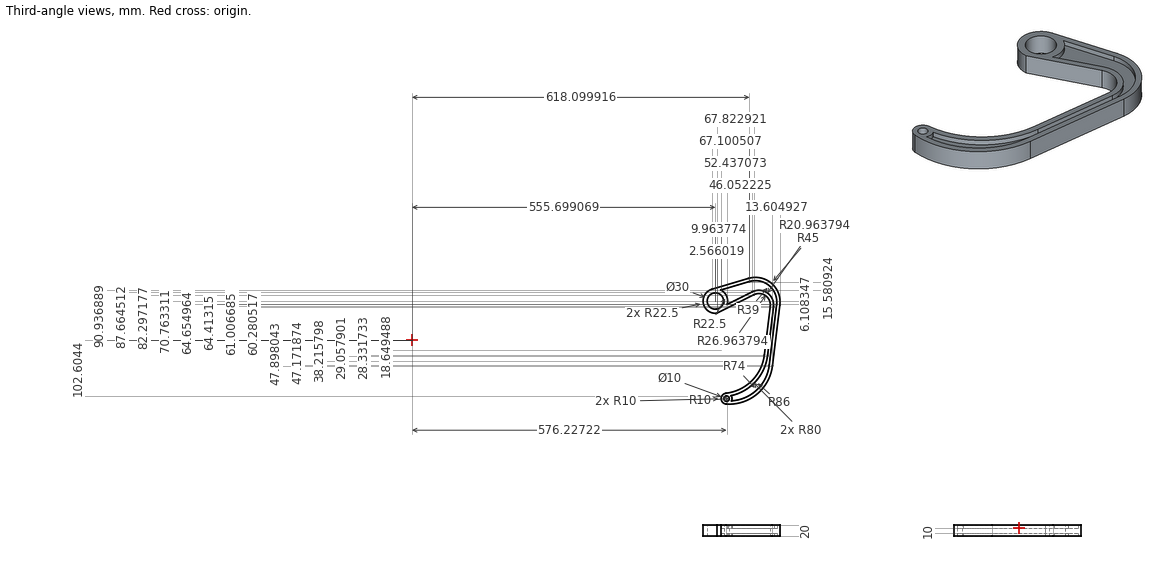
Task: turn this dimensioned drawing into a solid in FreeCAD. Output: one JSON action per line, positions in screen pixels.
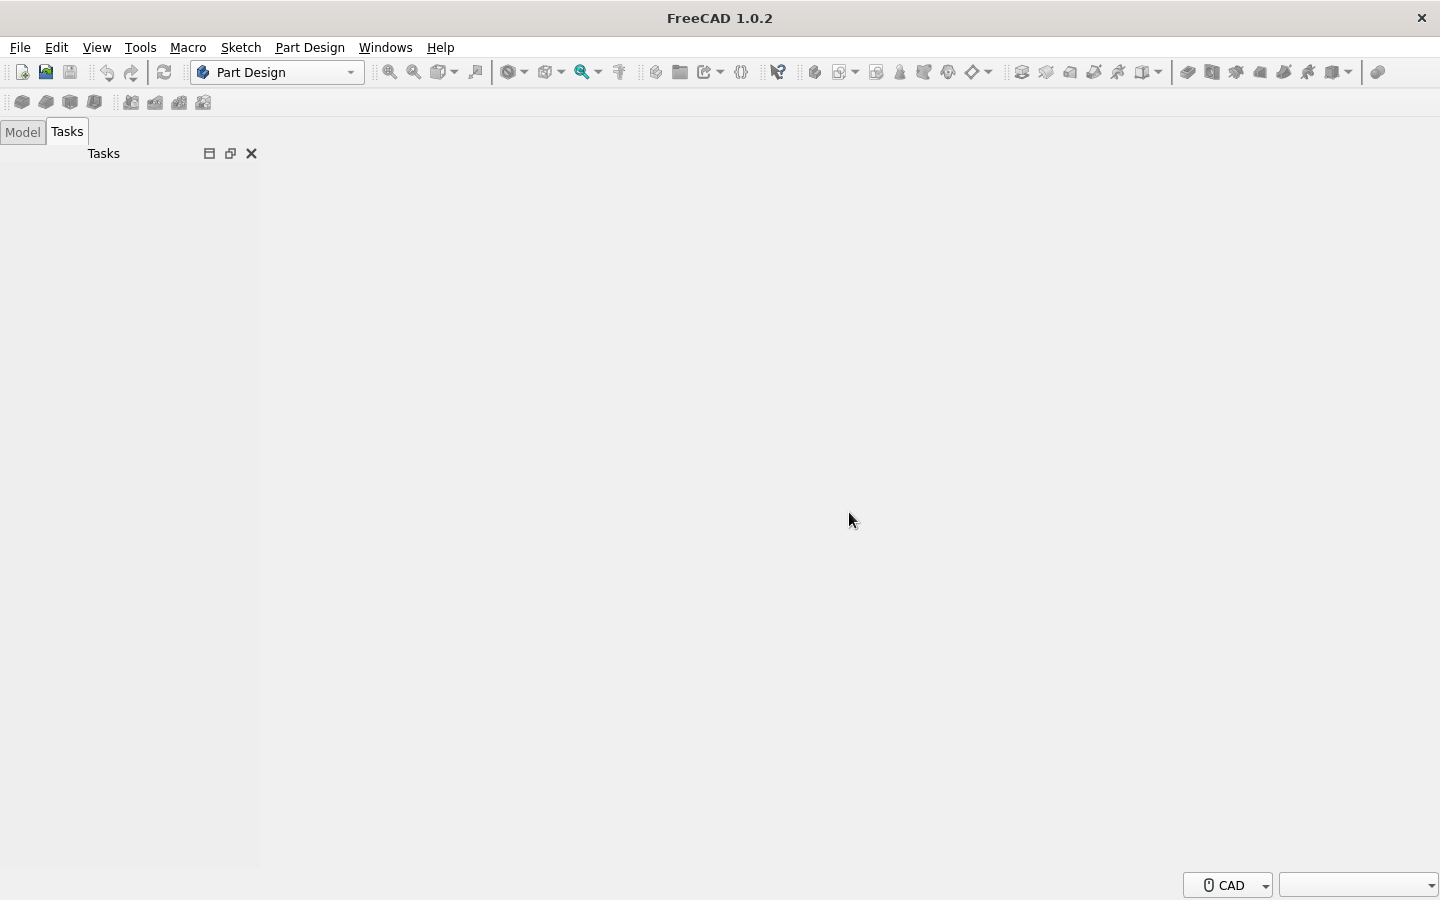
{"action": "left_click", "coordinate": [22, 72]}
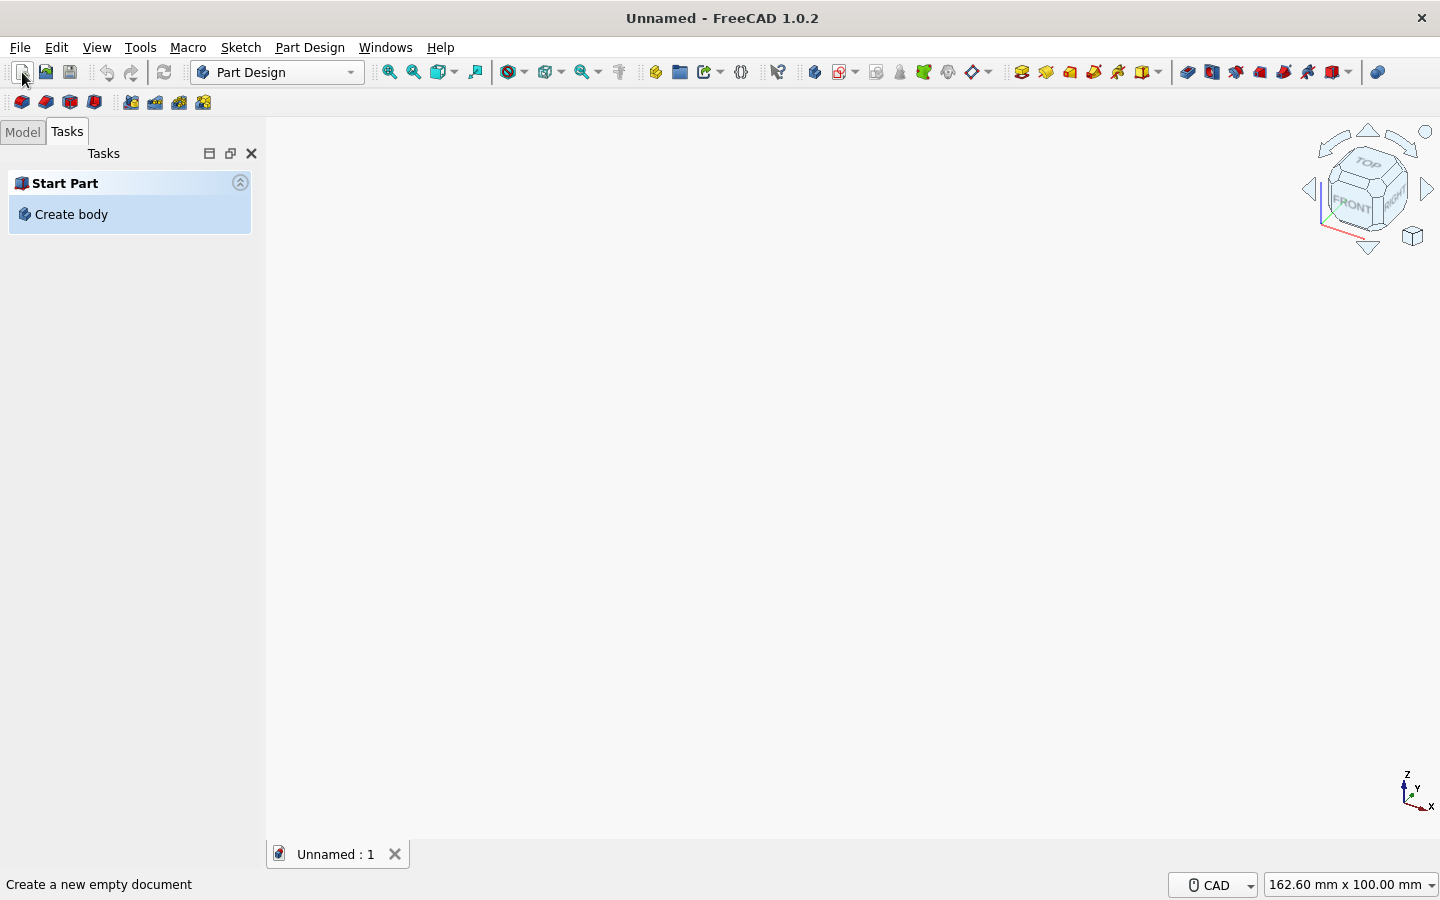
{"action": "left_click", "coordinate": [840, 72]}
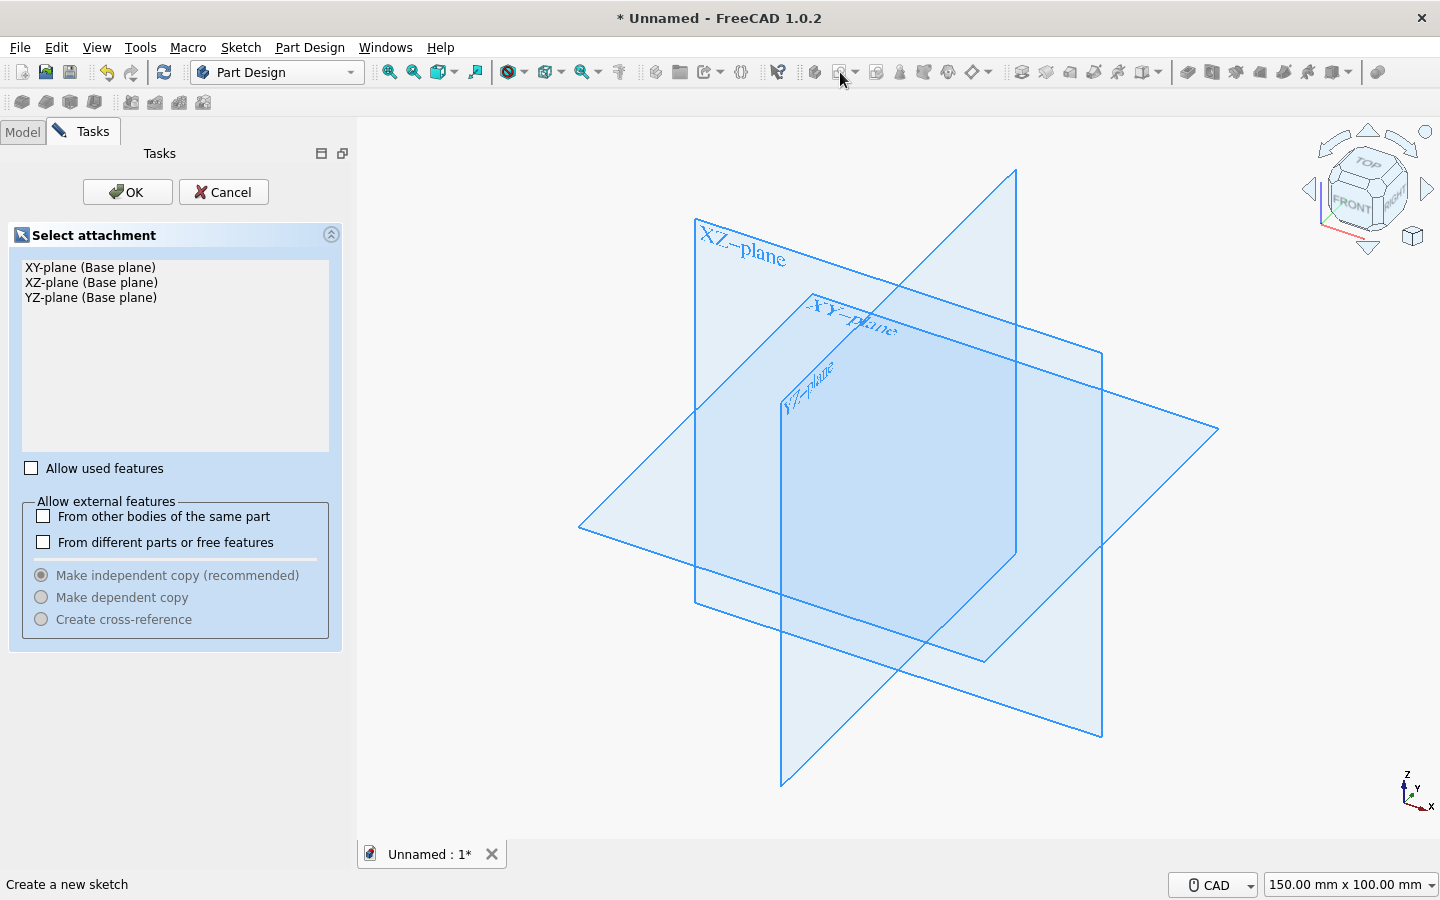
{"action": "left_click", "coordinate": [82, 268]}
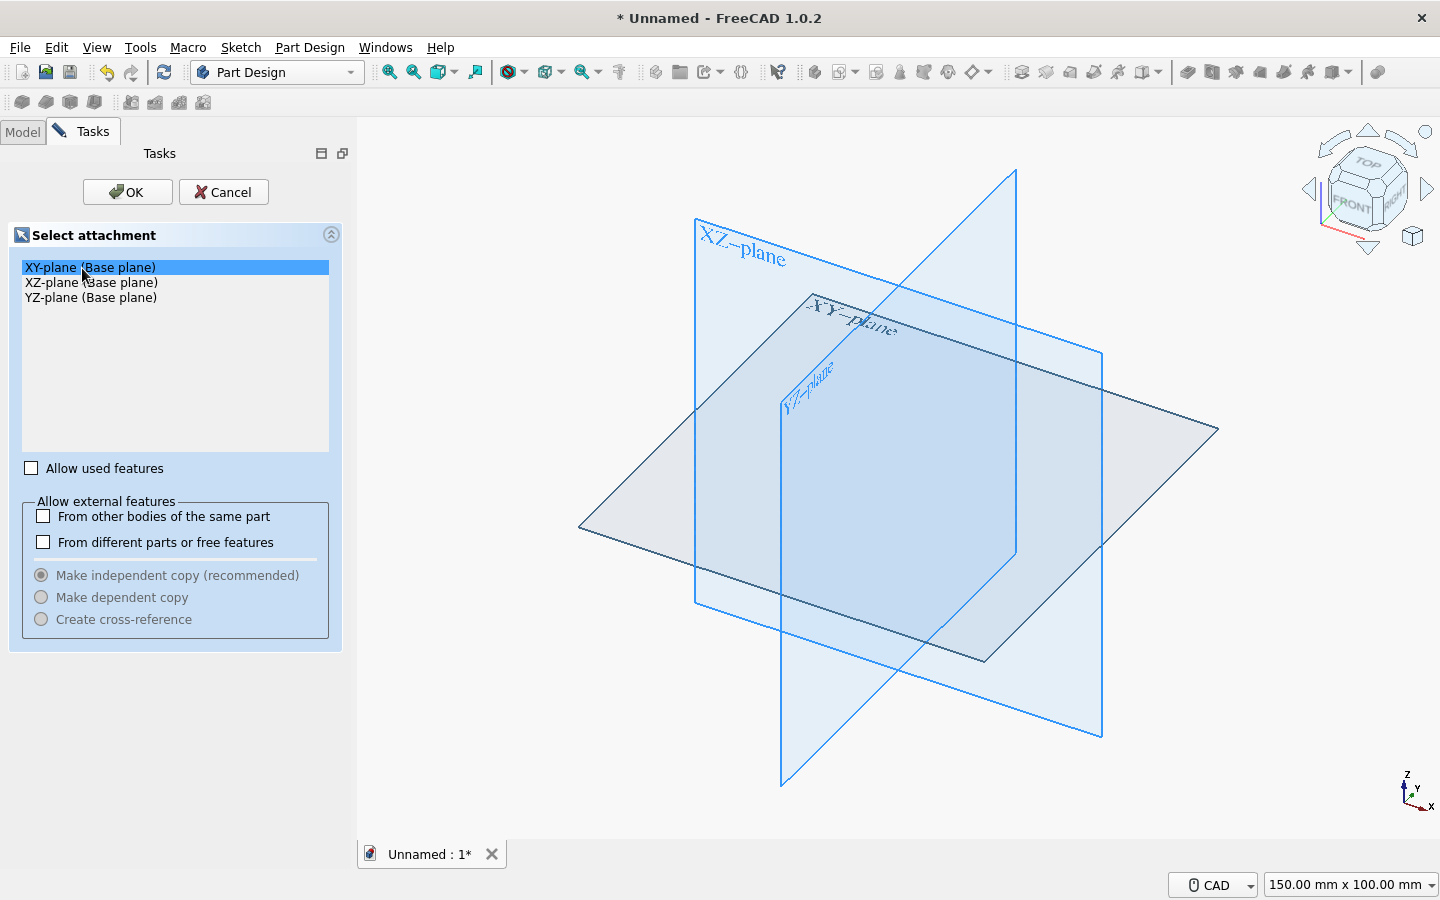
{"action": "left_click", "coordinate": [128, 192]}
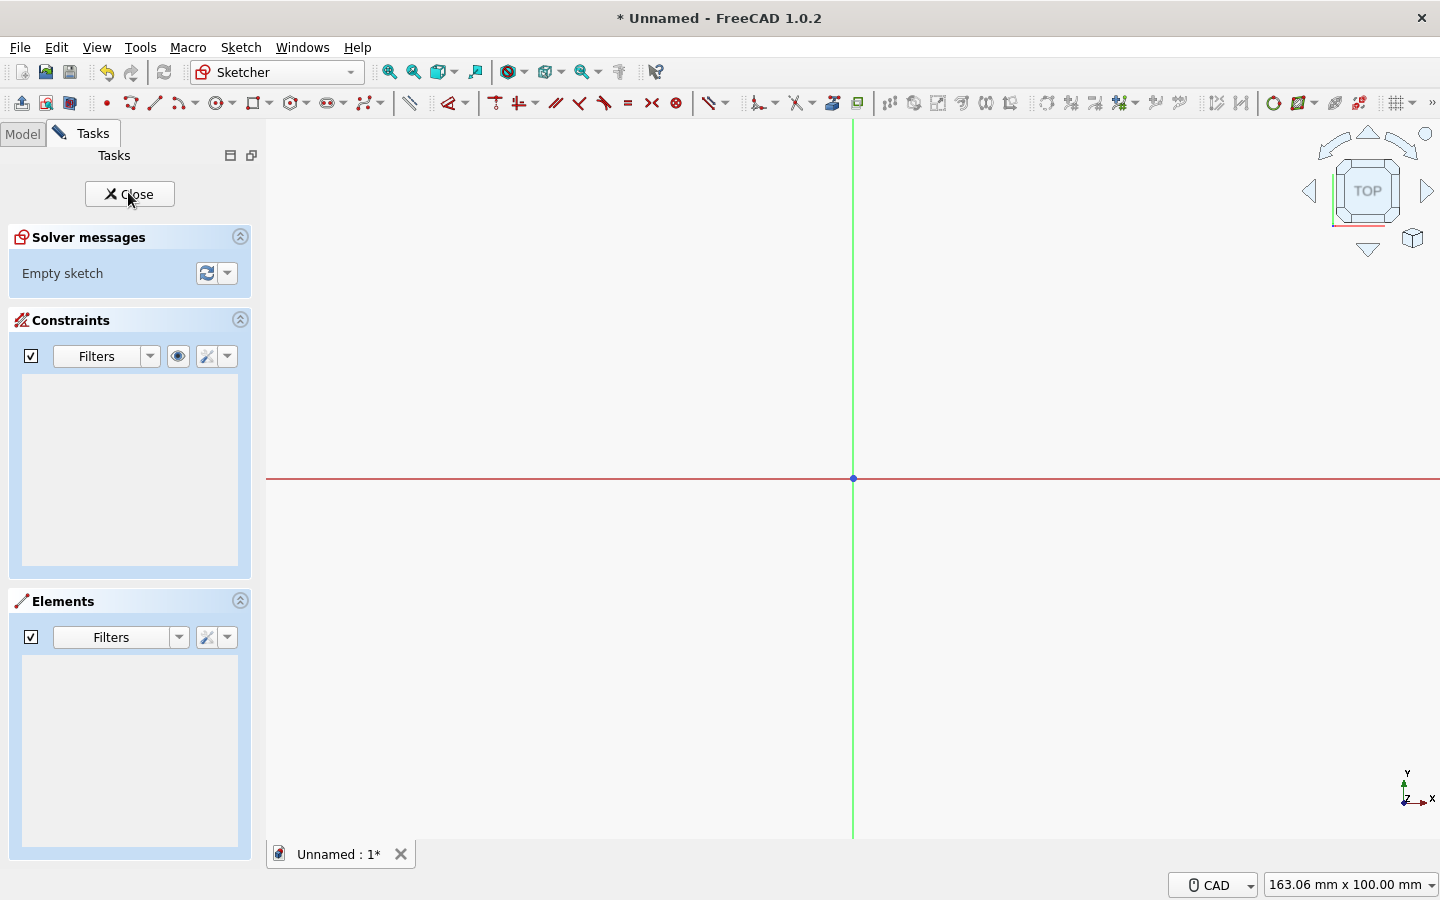
{"action": "scroll", "coordinate": [294, 475], "scroll_direction": "down", "scroll_amount": 9}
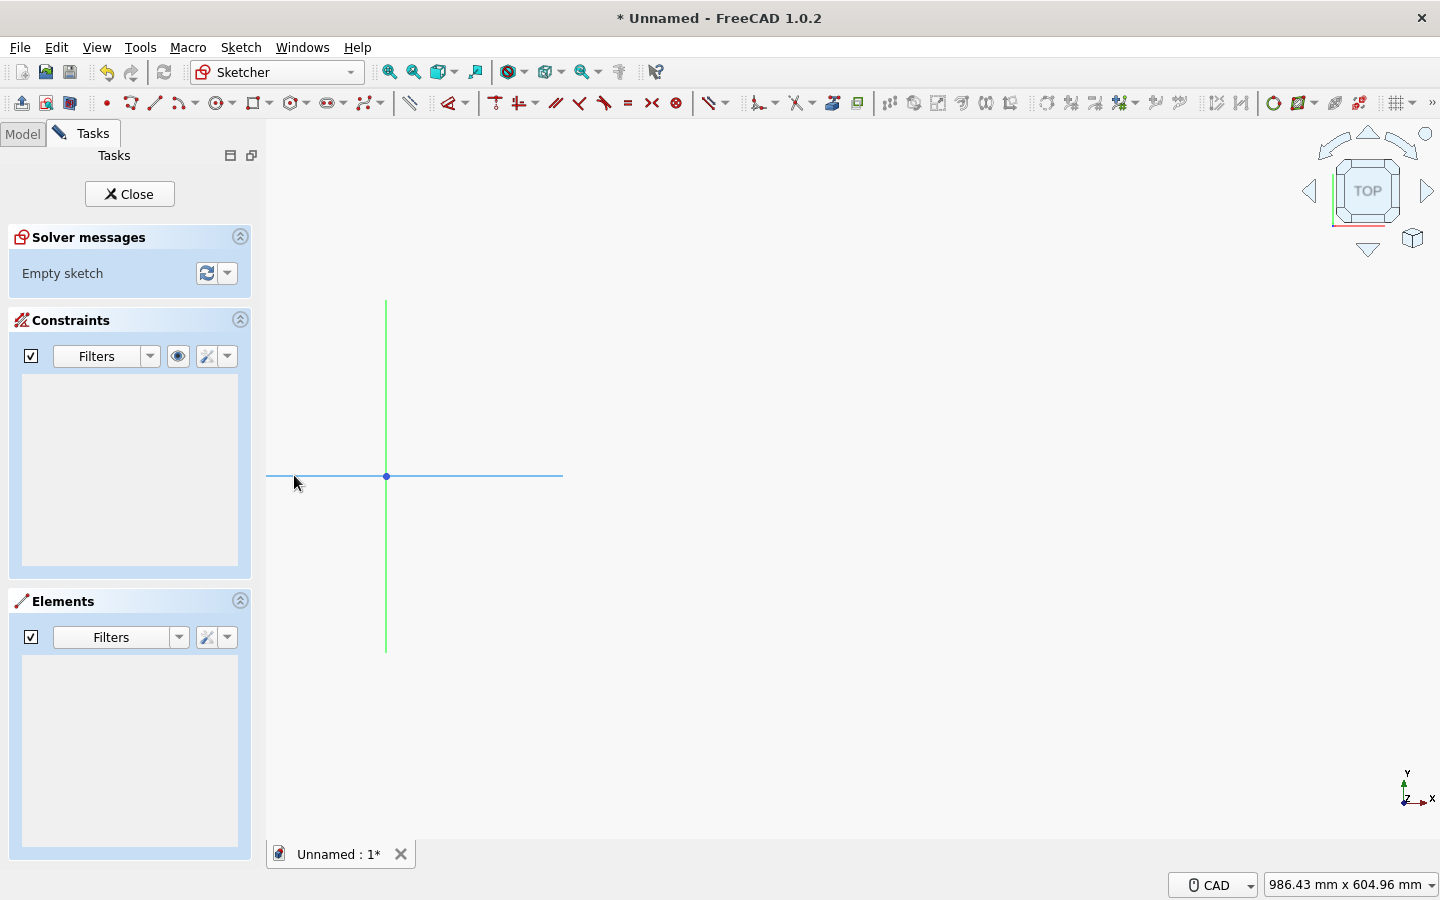
{"action": "scroll", "coordinate": [1275, 480], "scroll_direction": "up", "scroll_amount": 3}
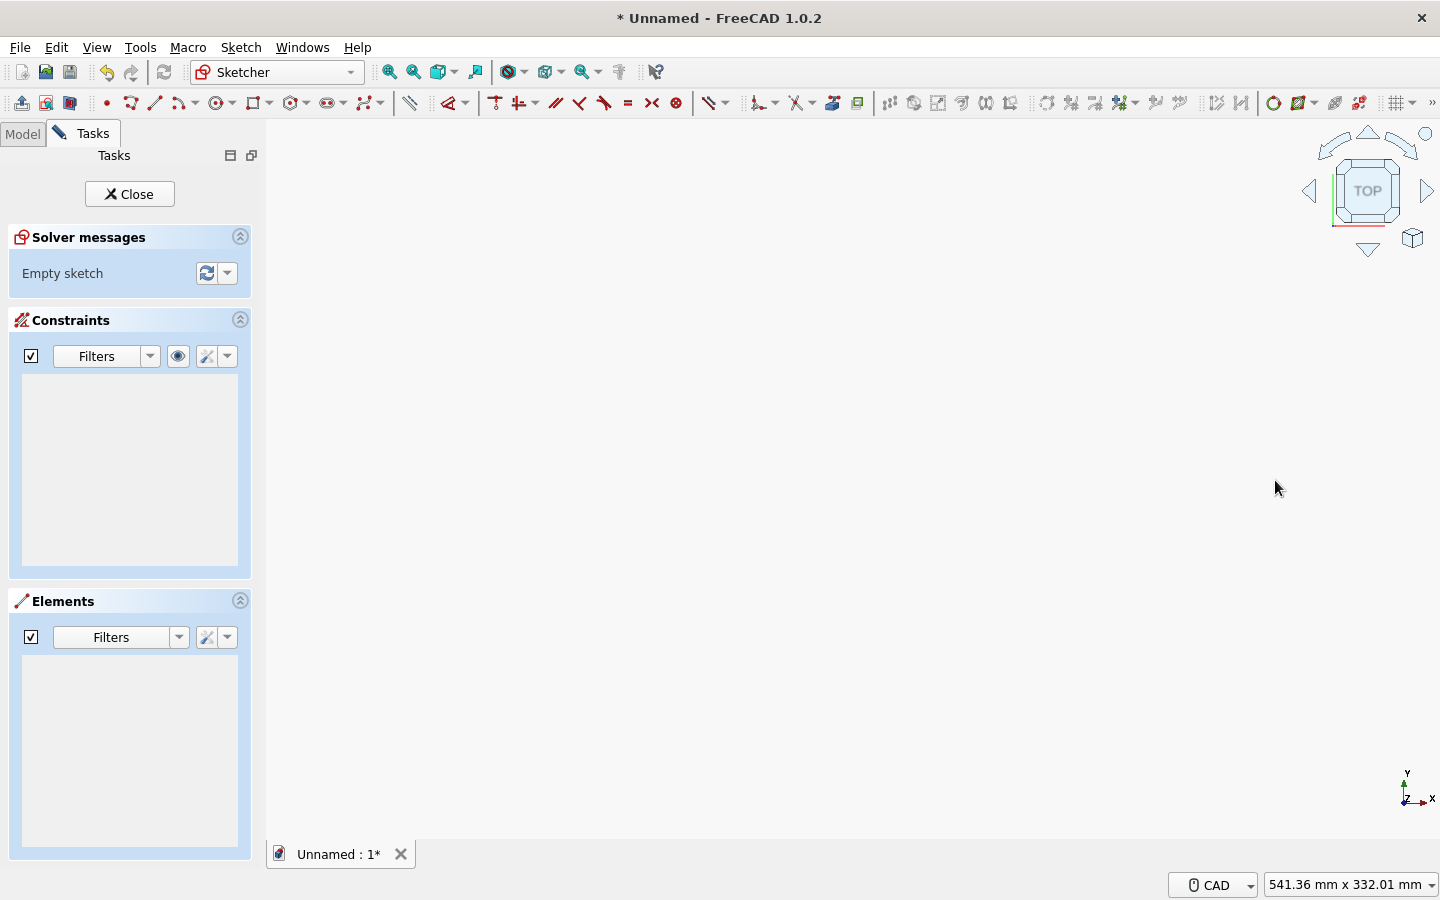
{"action": "left_click", "coordinate": [156, 104]}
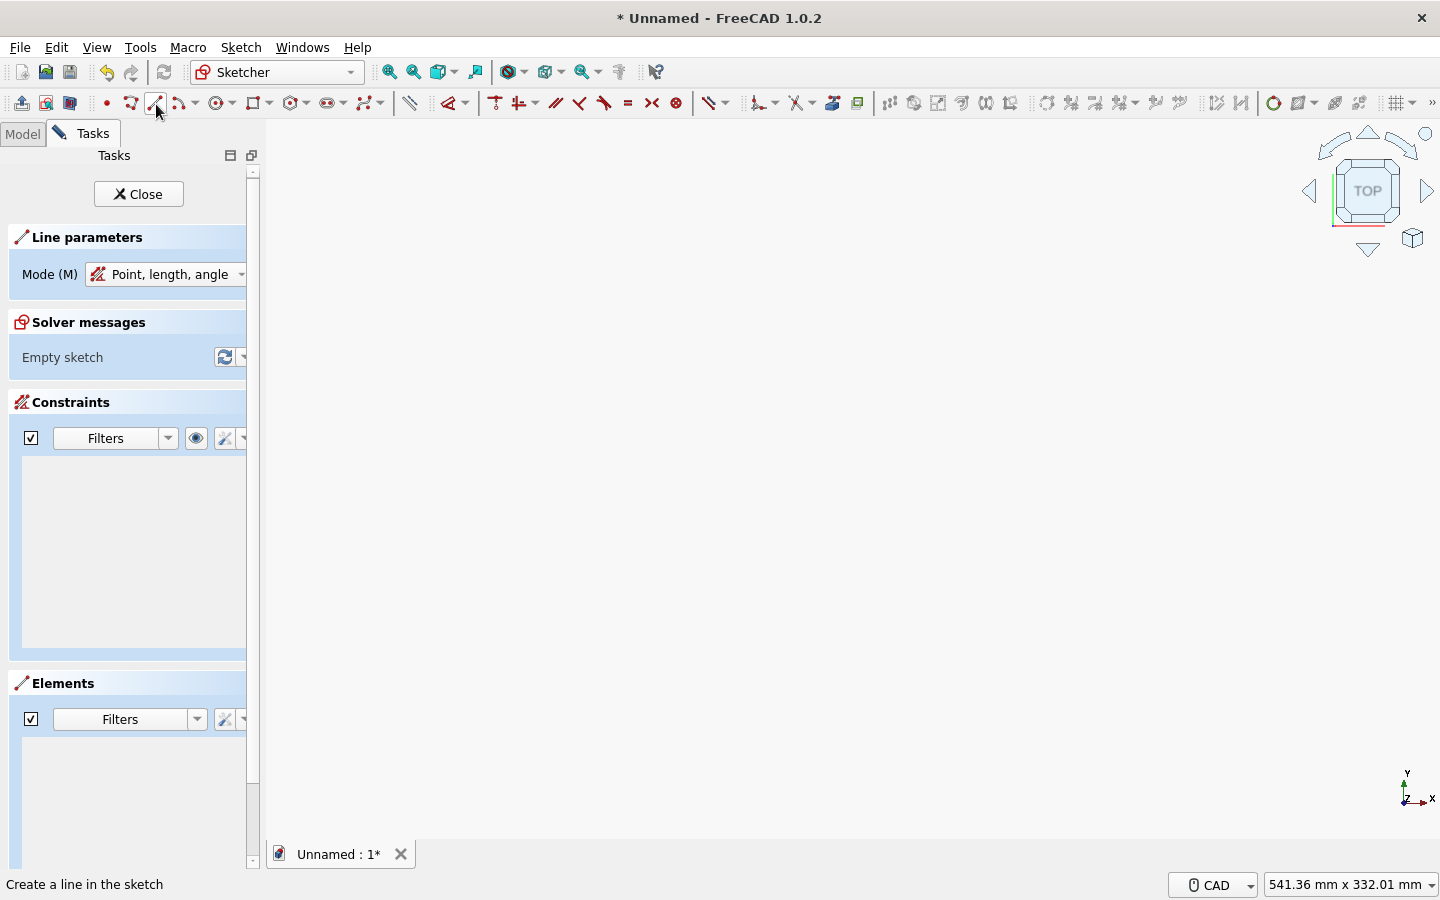
{"action": "left_click", "coordinate": [996, 241]}
{"action": "left_click", "coordinate": [882, 275]}